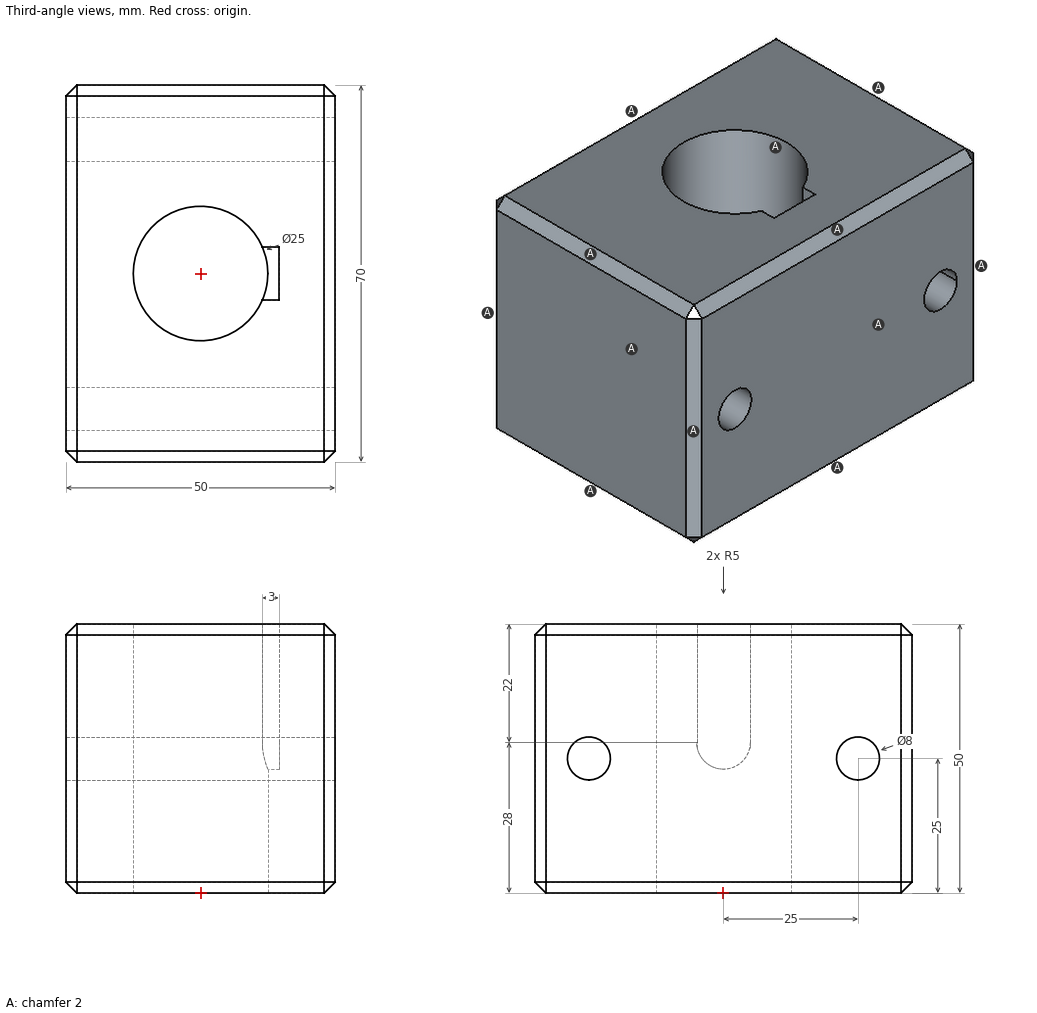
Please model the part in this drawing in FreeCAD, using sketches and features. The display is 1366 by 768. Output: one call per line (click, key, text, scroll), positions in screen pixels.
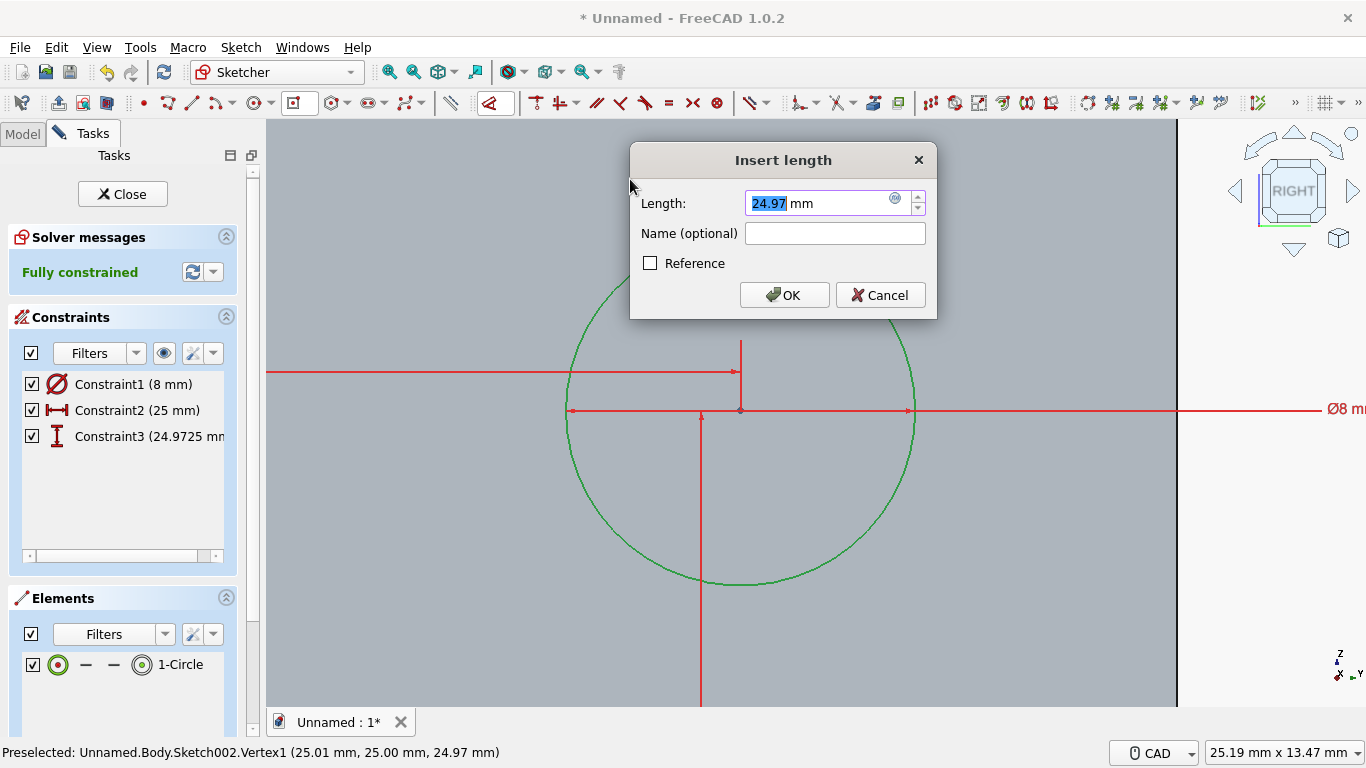
text(25)
key(Return)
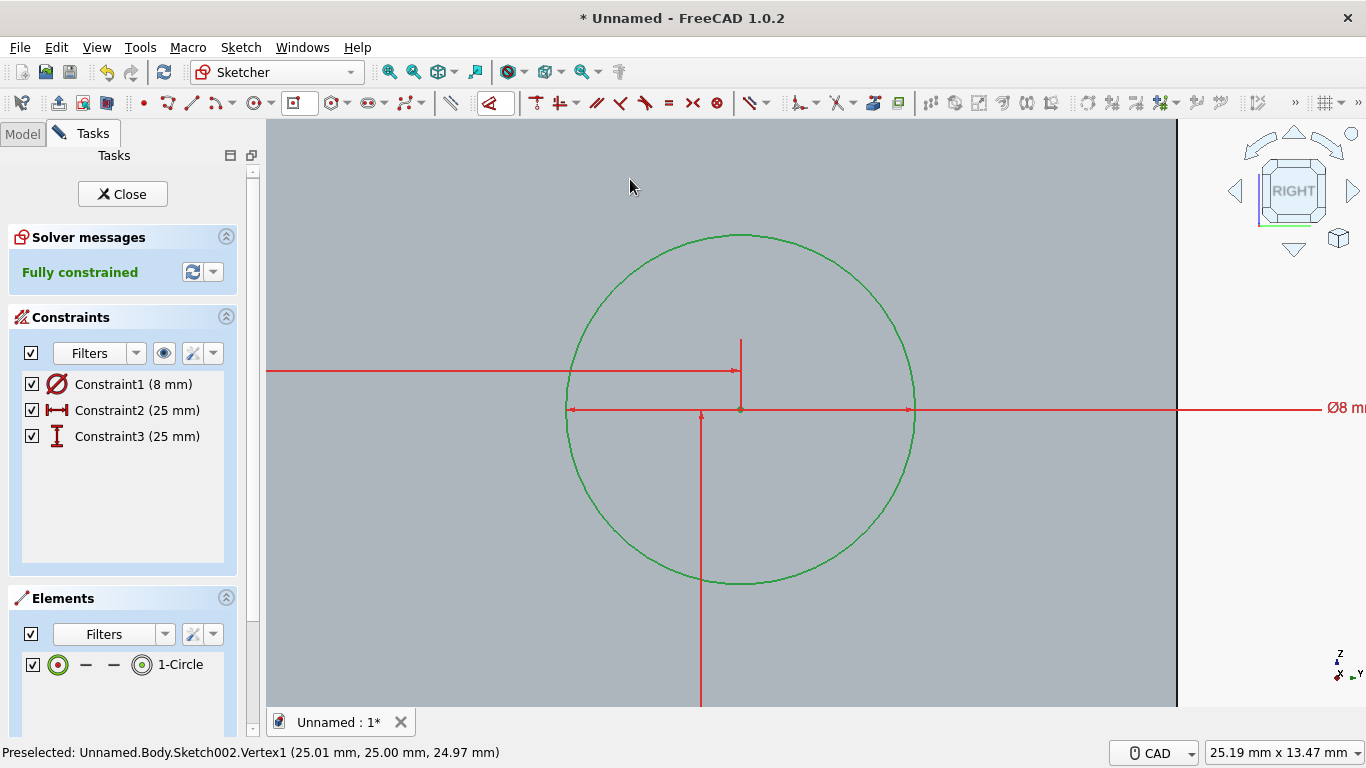
click(123, 194)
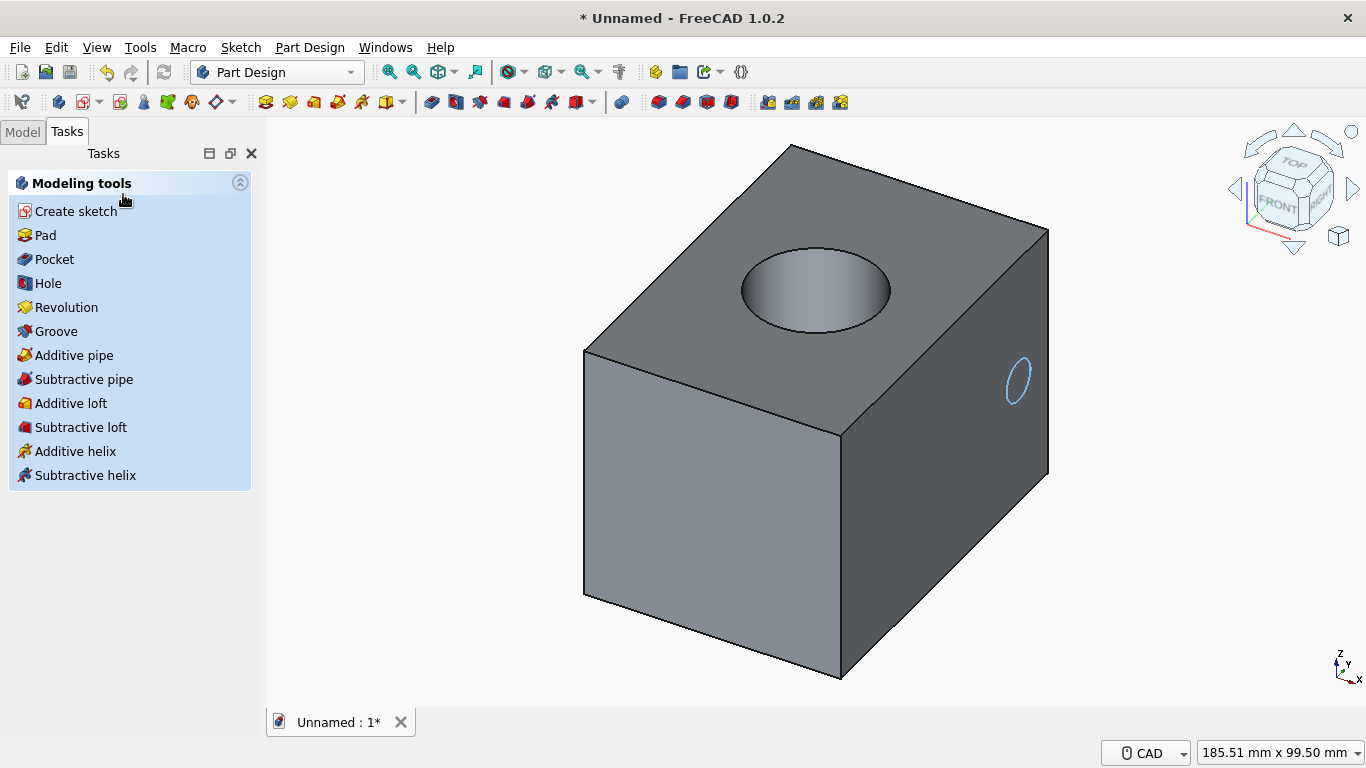
click(432, 102)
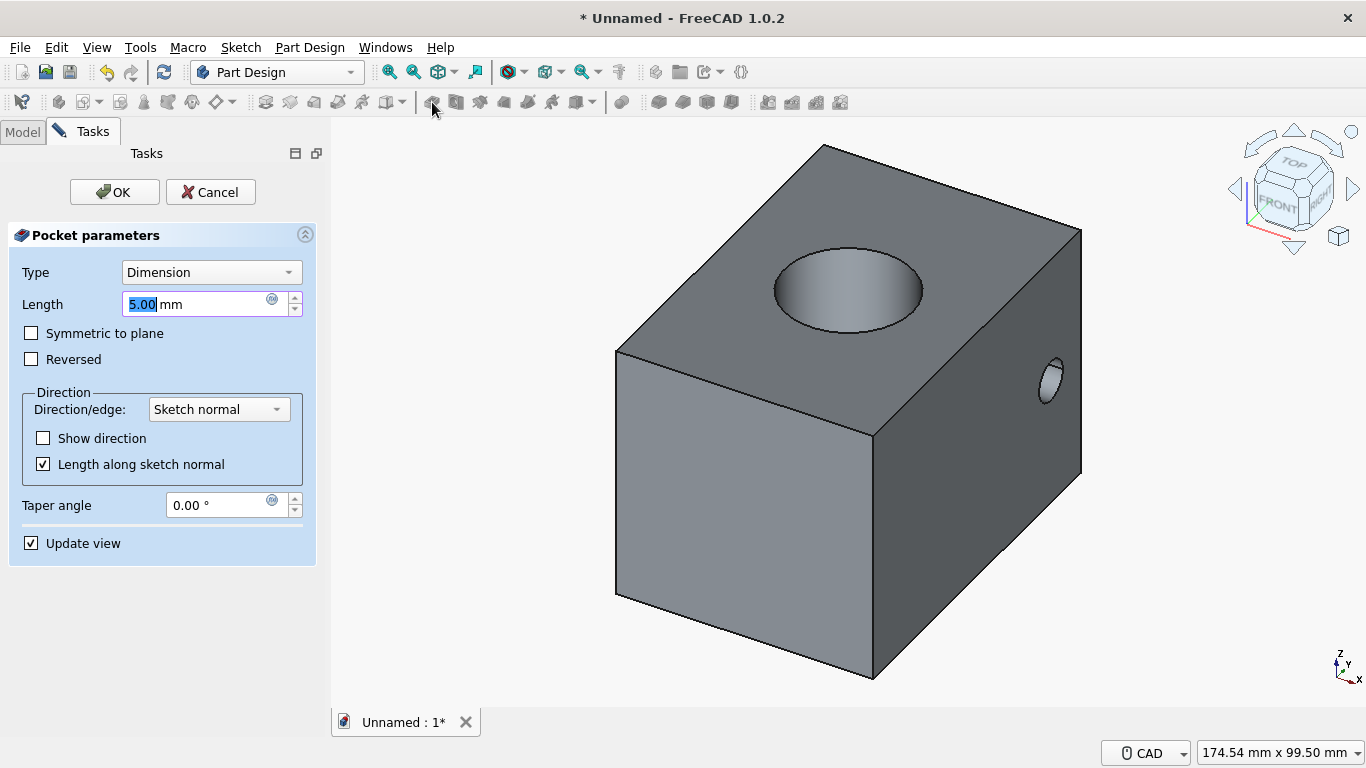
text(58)
key(Tab)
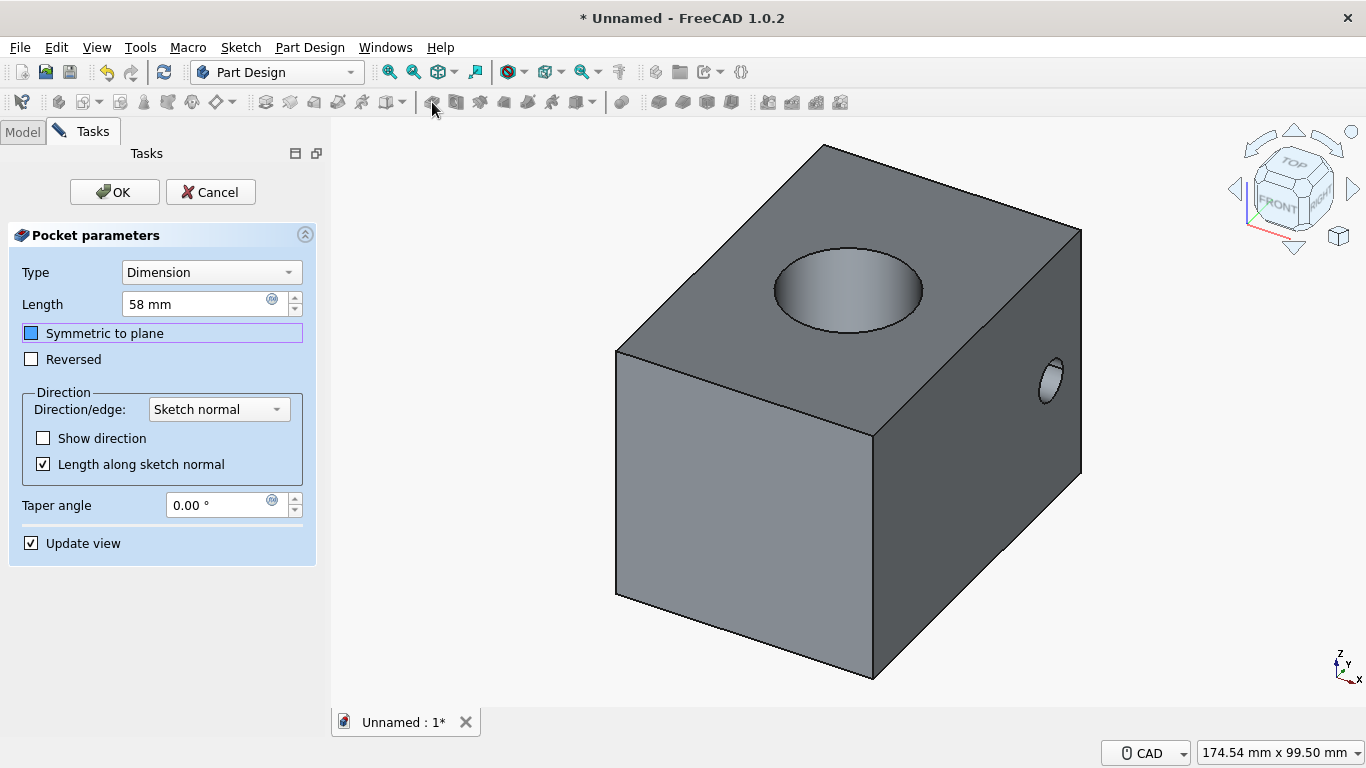
click(115, 192)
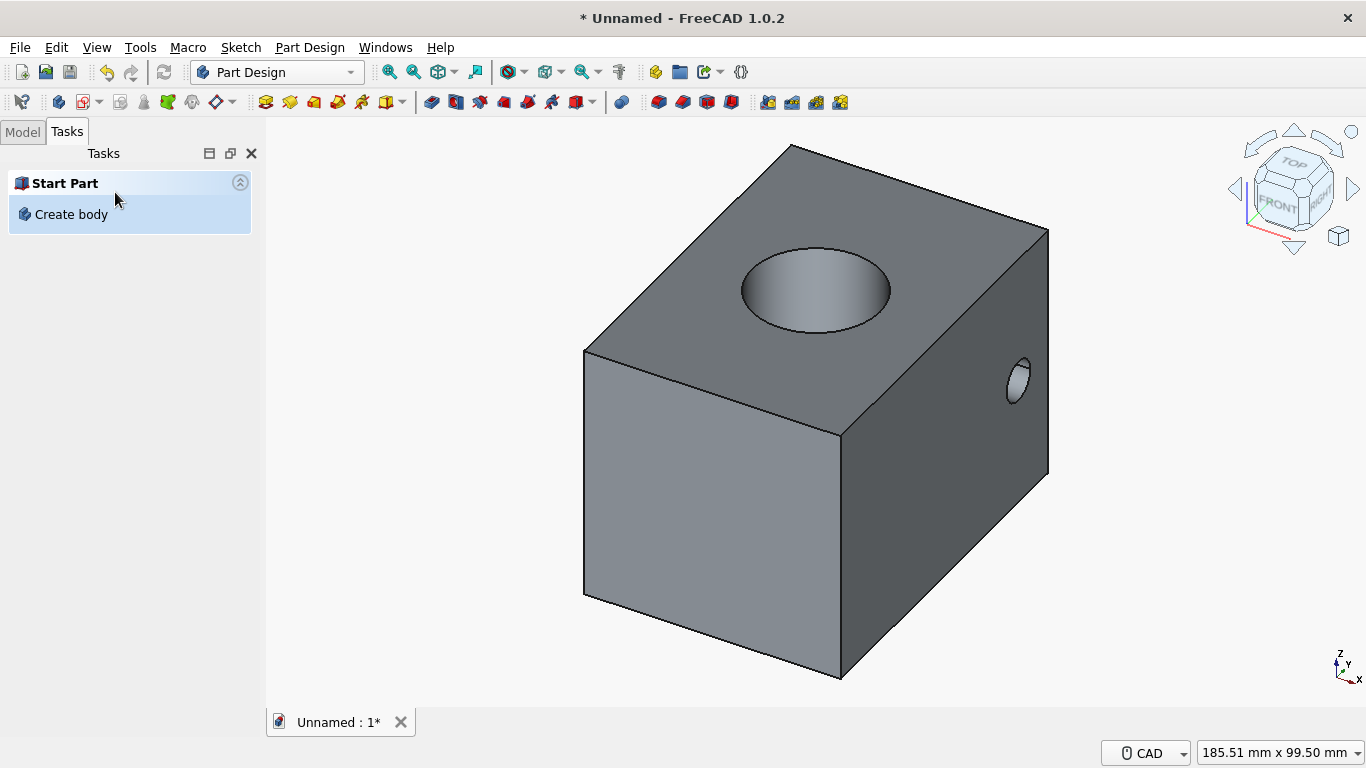
click(23, 131)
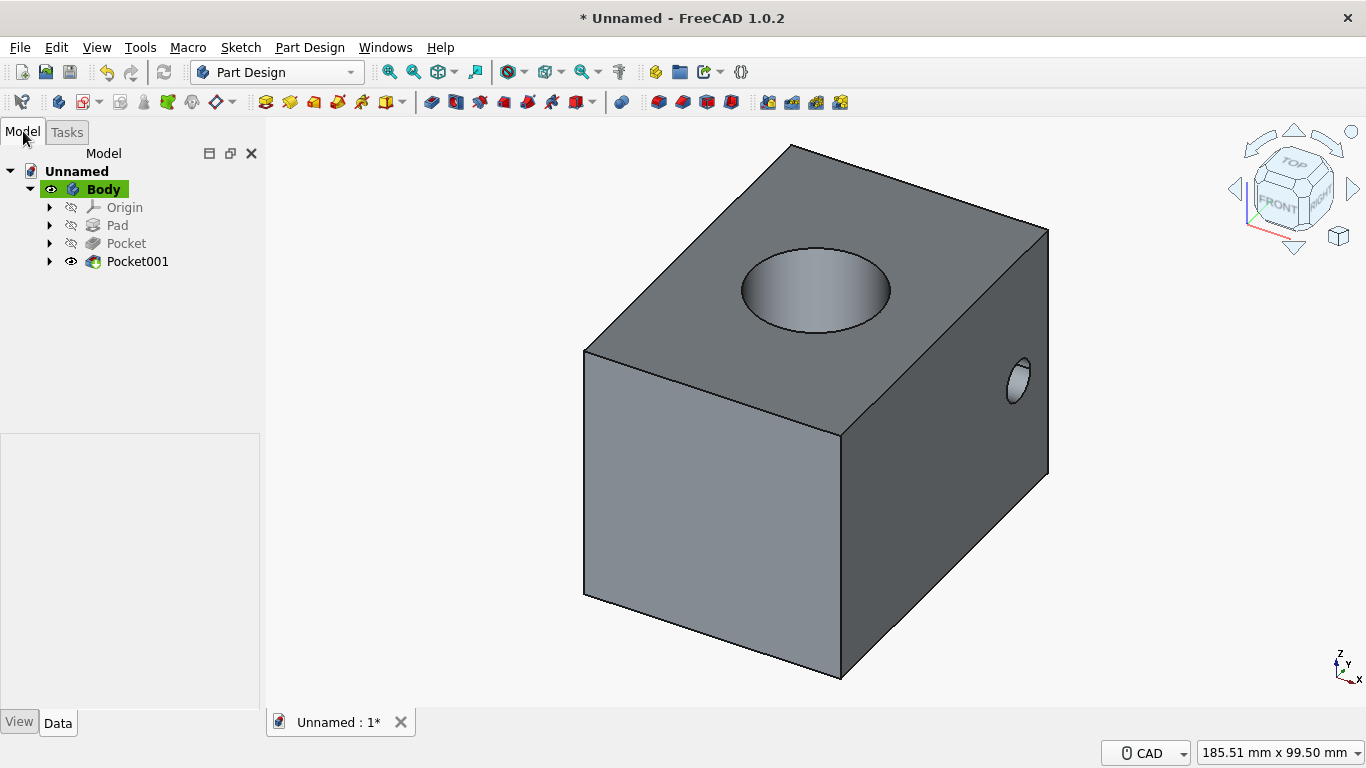
click(116, 261)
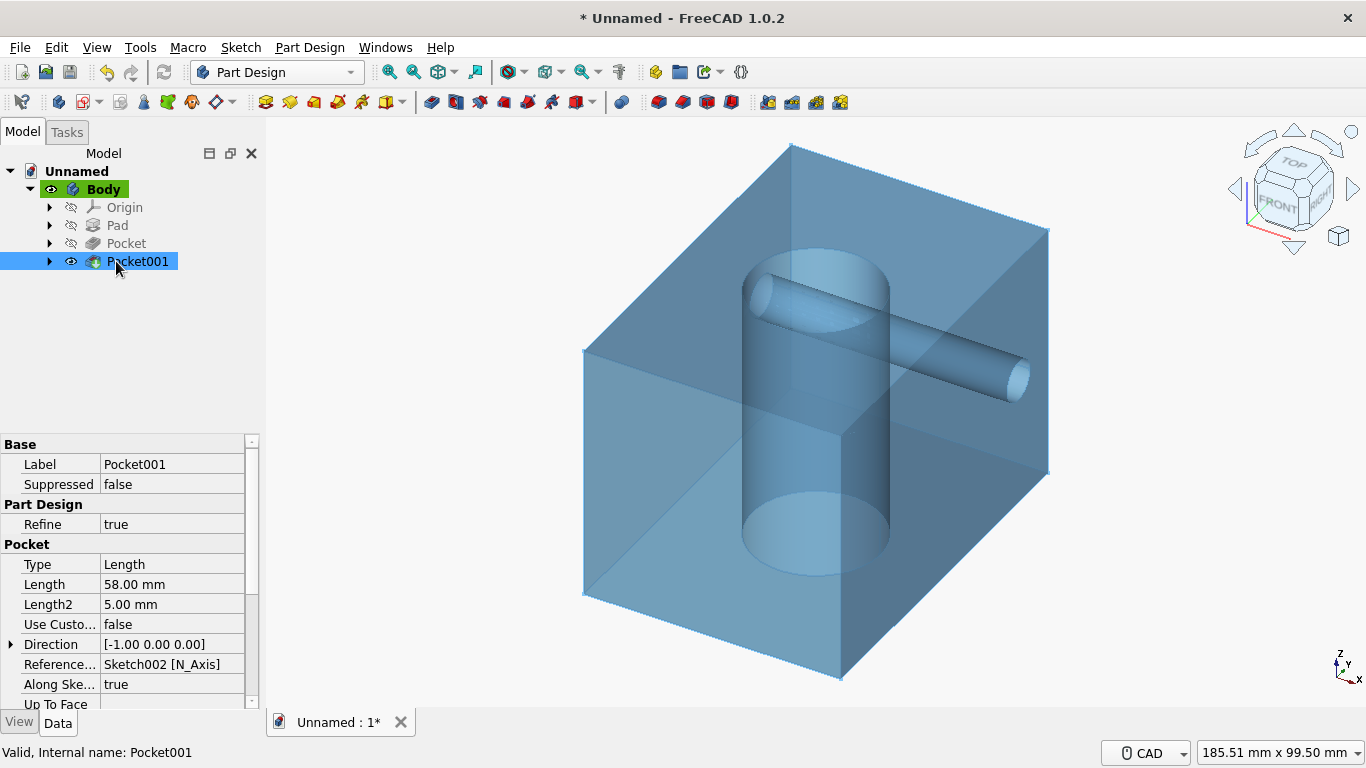
click(768, 102)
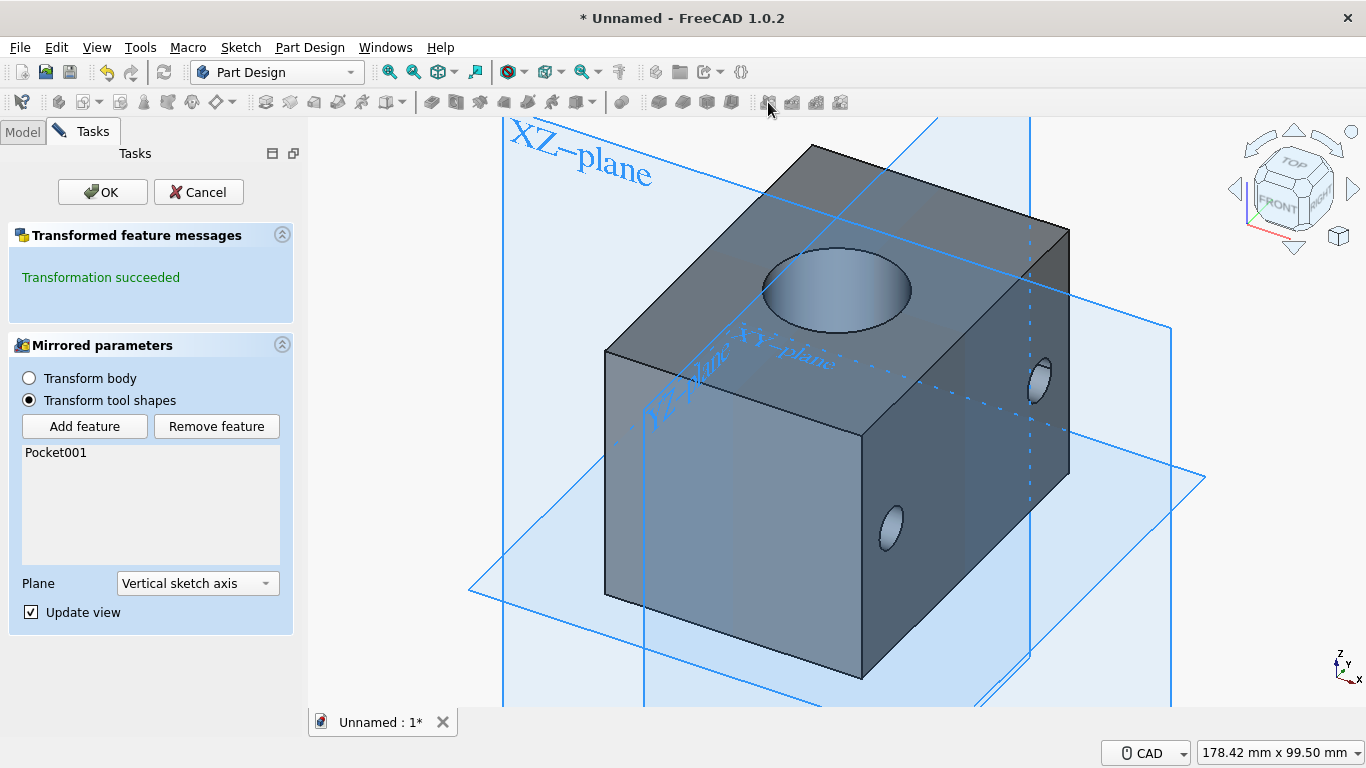
click(198, 584)